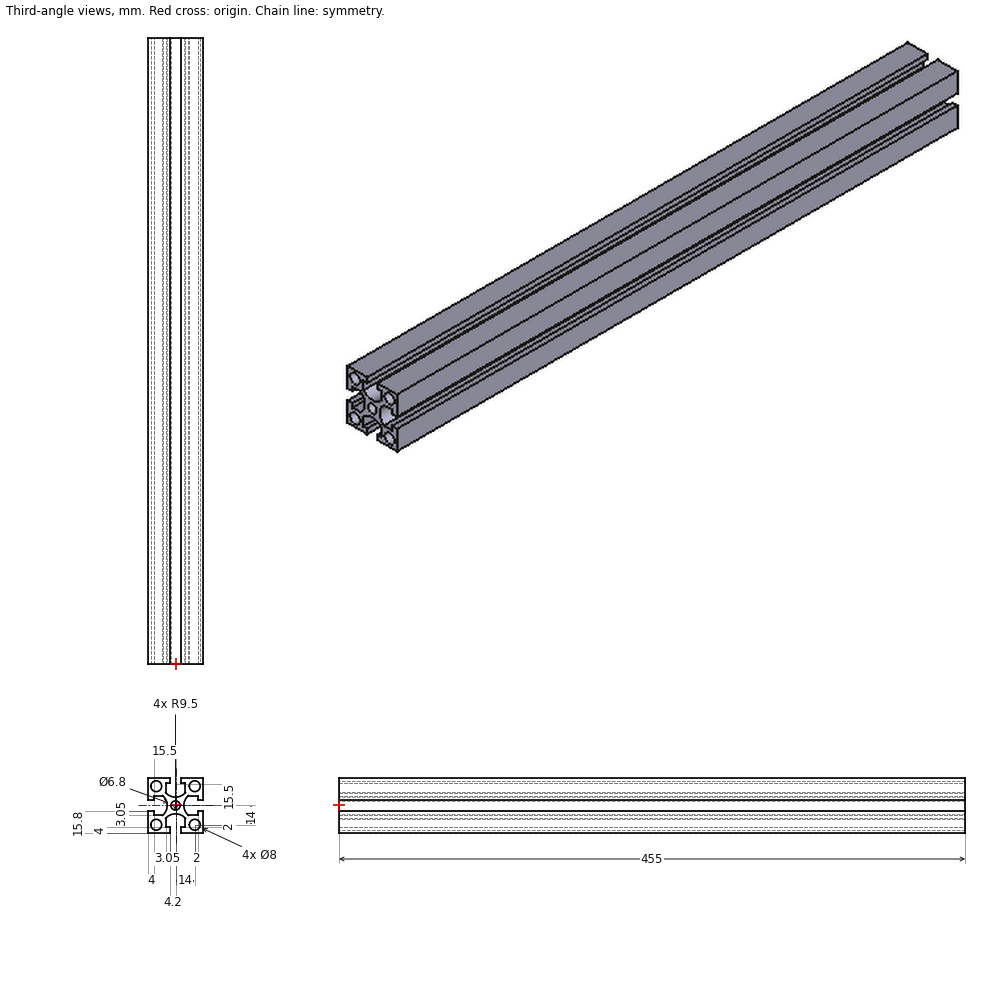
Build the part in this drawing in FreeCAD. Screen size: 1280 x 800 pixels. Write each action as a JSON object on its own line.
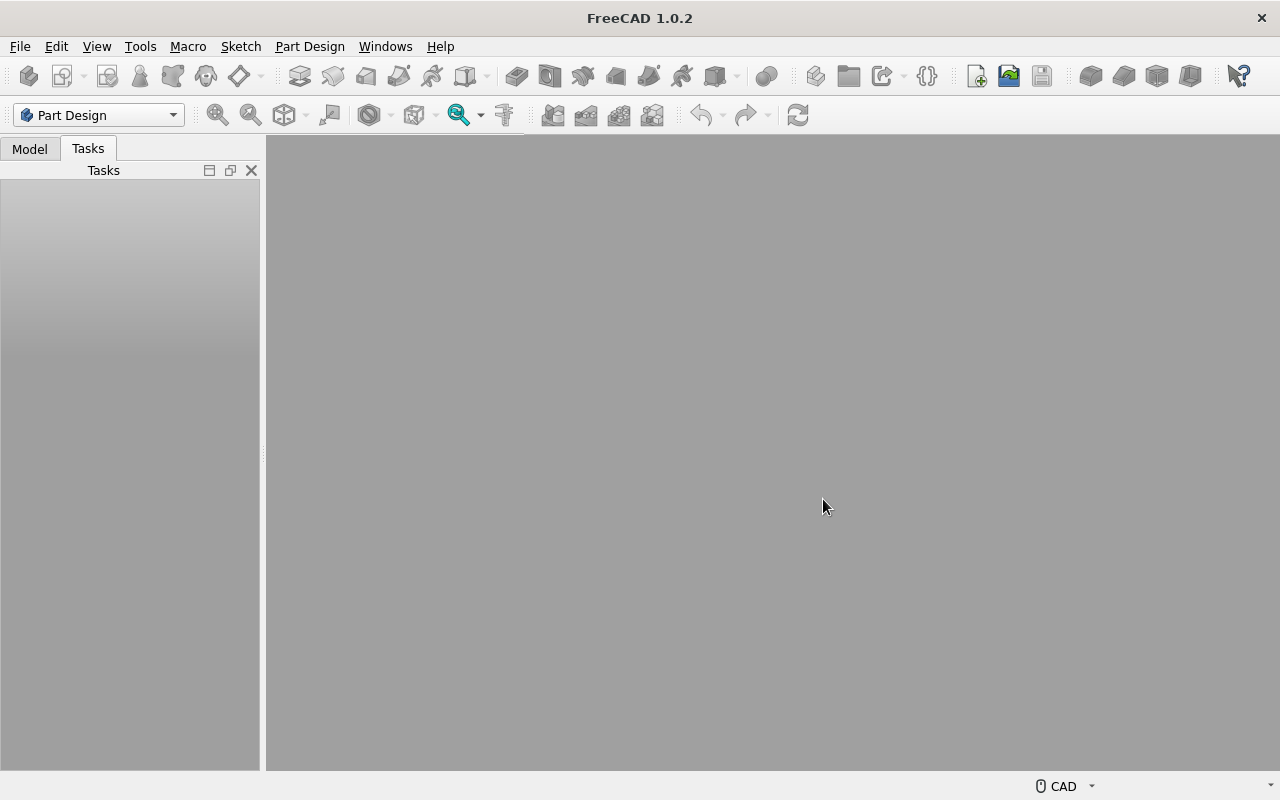
{"action": "left_click", "coordinate": [976, 76]}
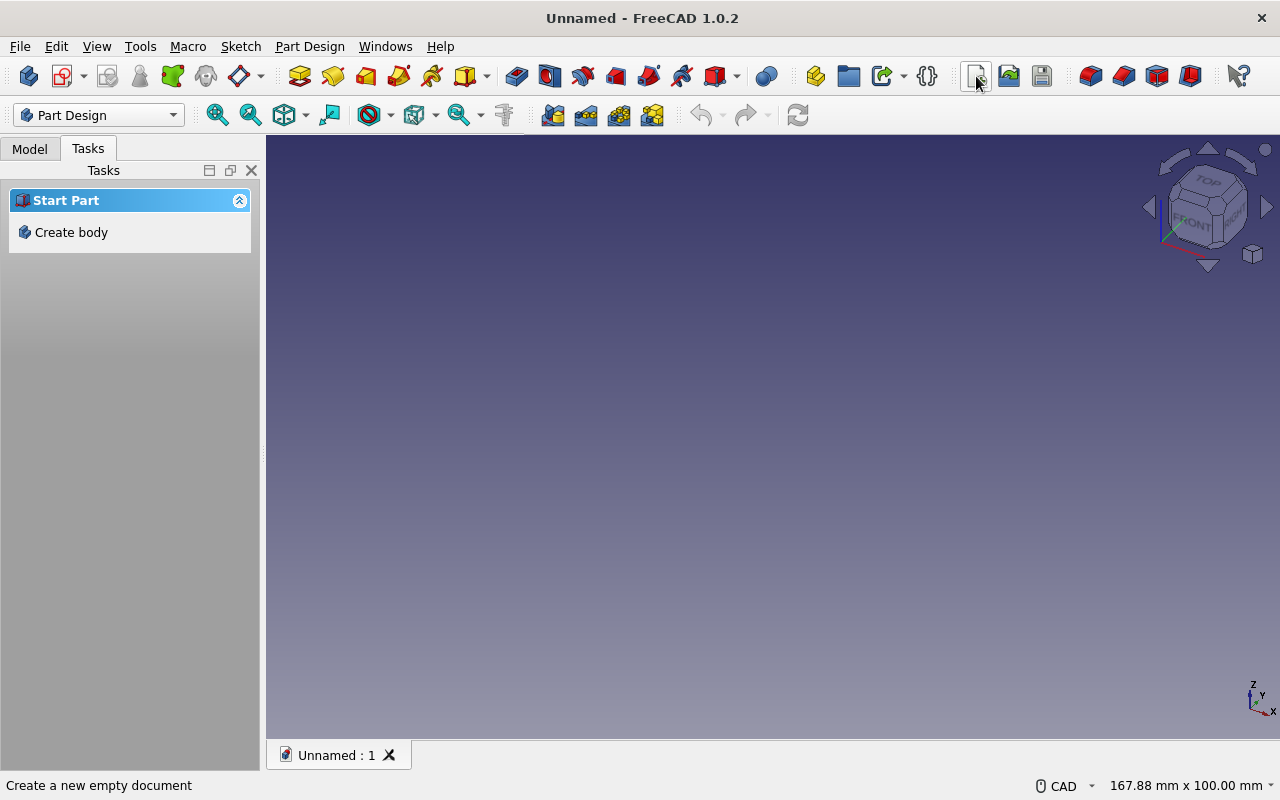
{"action": "left_click", "coordinate": [62, 76]}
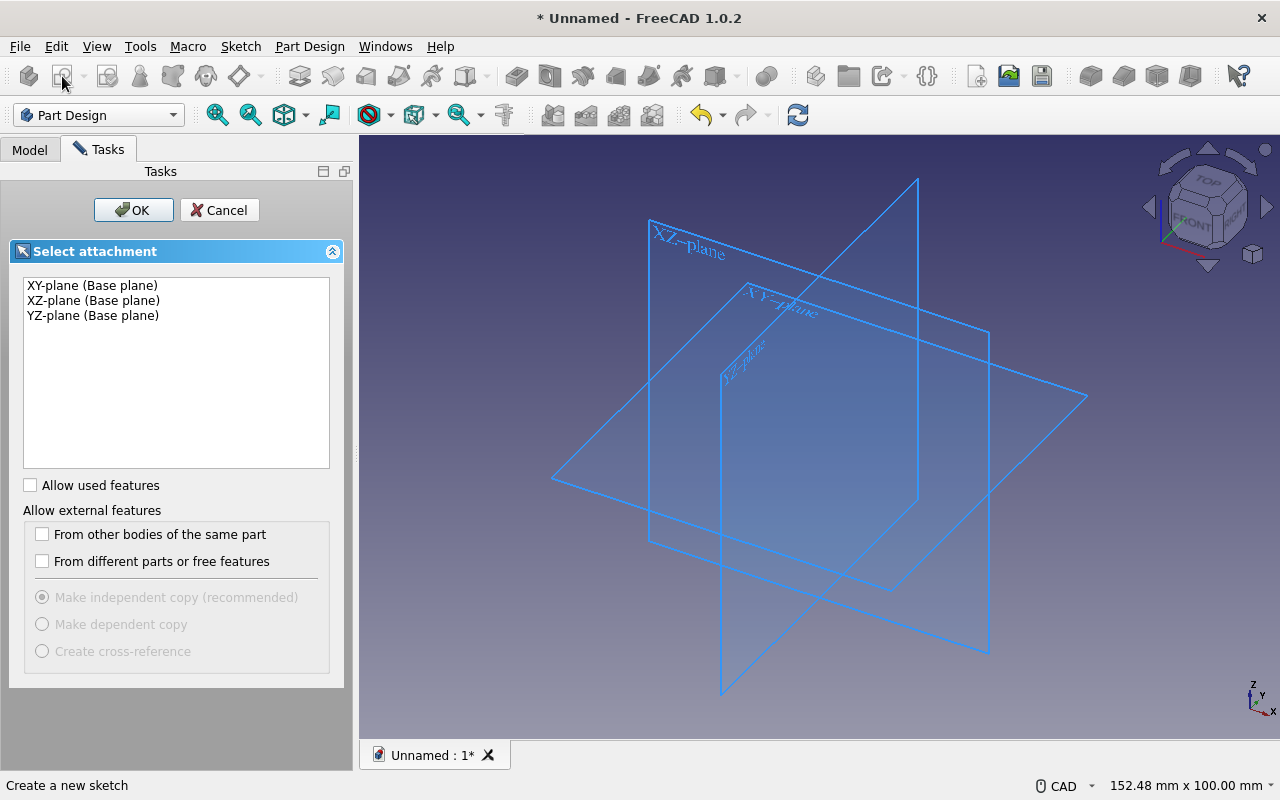
{"action": "left_click", "coordinate": [84, 300]}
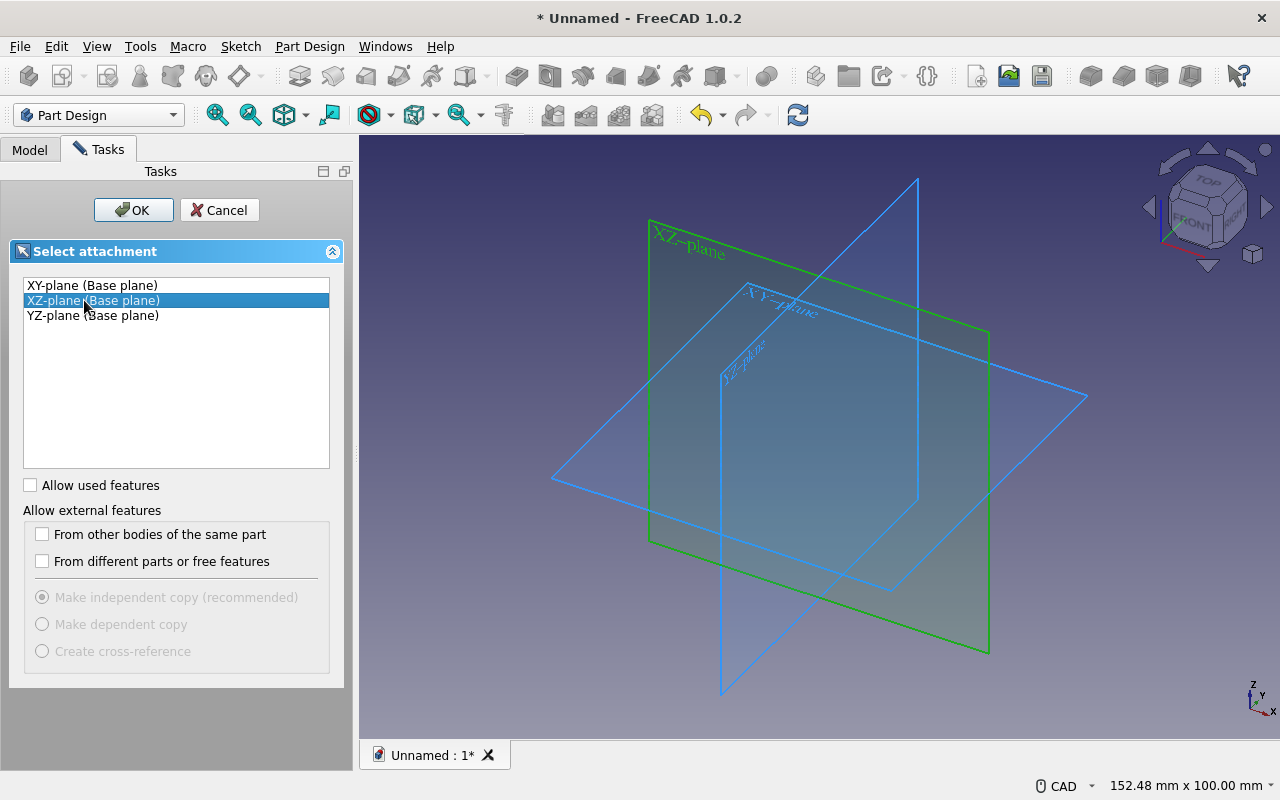
{"action": "left_click", "coordinate": [134, 210]}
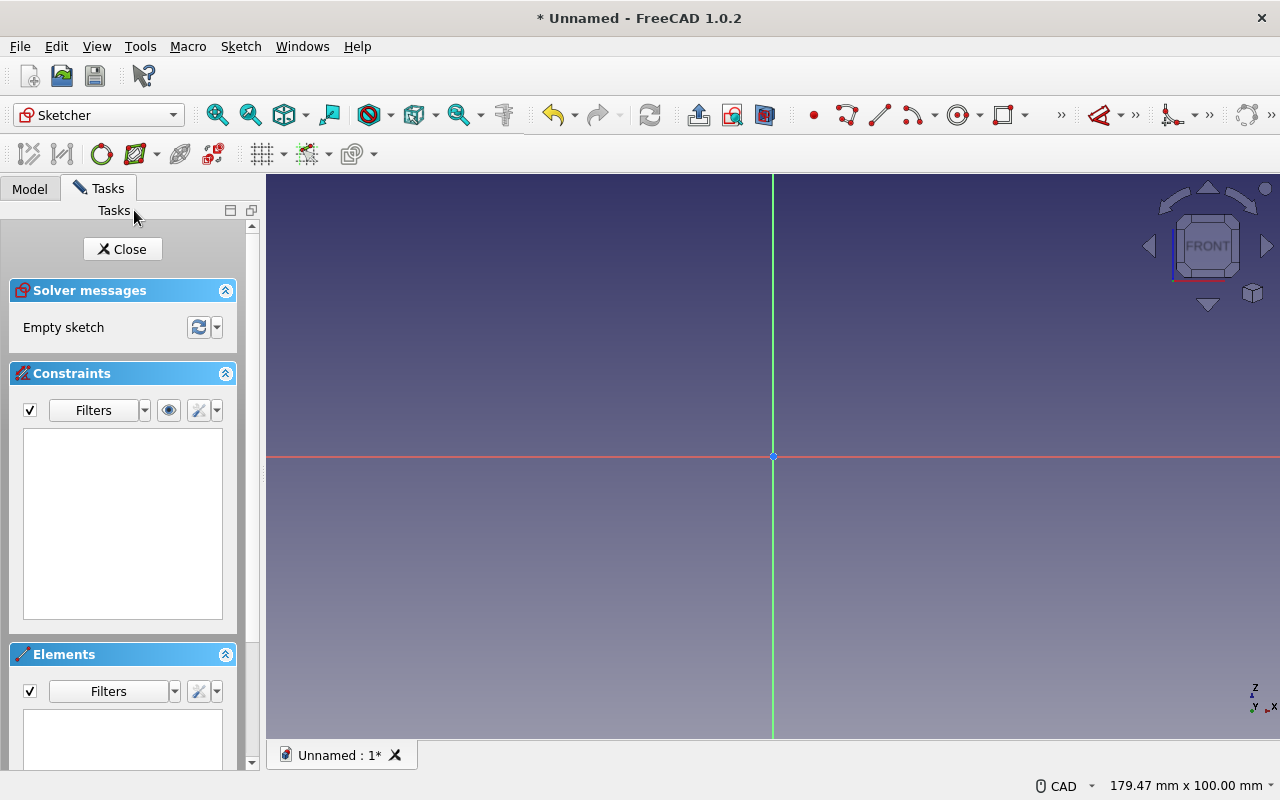
{"action": "scroll", "coordinate": [912, 456], "scroll_direction": "up", "scroll_amount": 2}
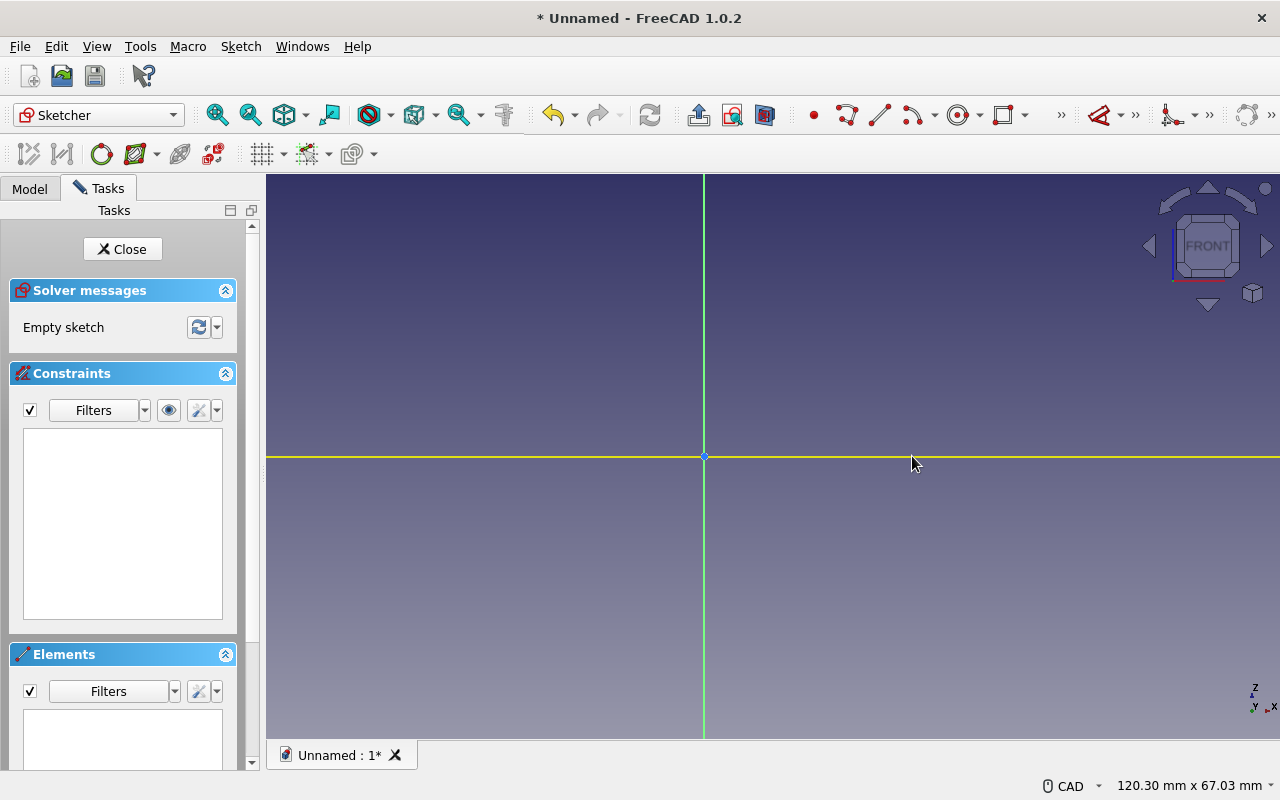
{"action": "left_click", "coordinate": [847, 116]}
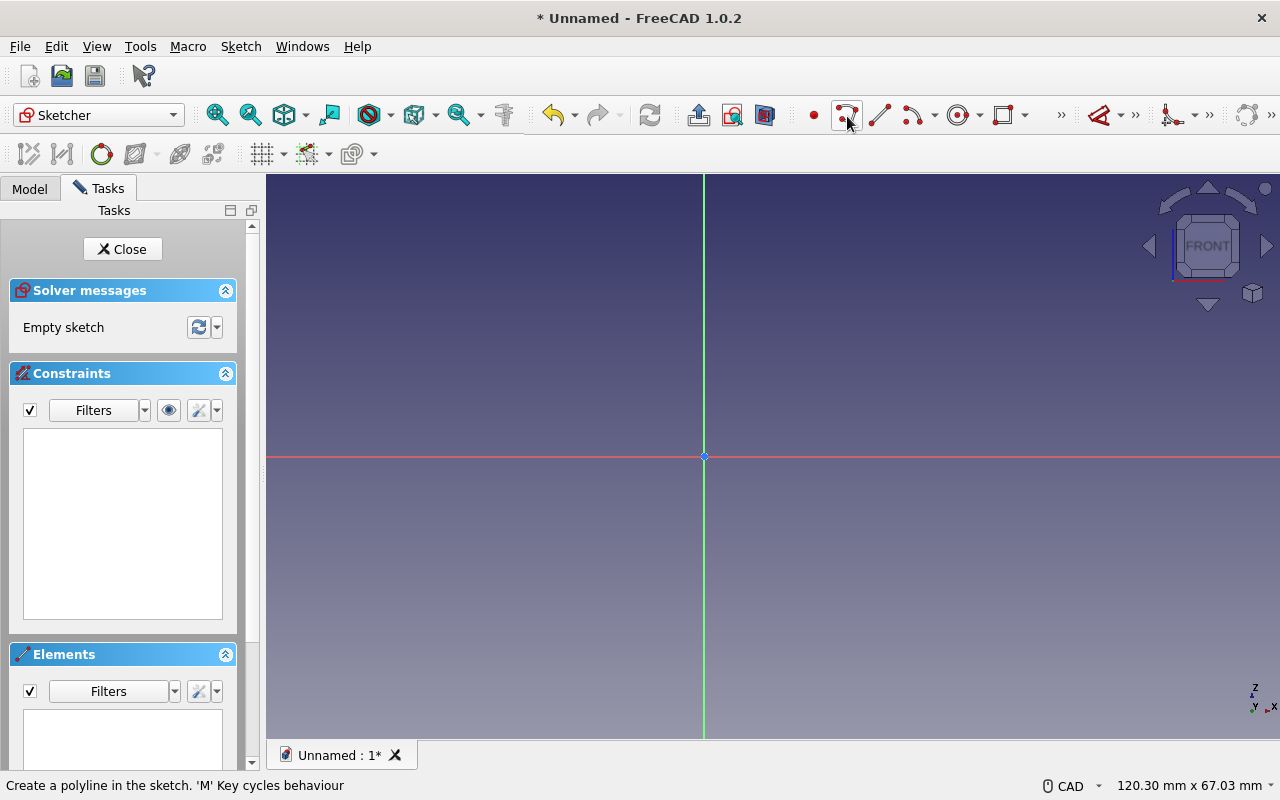
{"action": "left_click", "coordinate": [643, 535]}
{"action": "left_click", "coordinate": [643, 591]}
{"action": "left_click", "coordinate": [669, 591]}
{"action": "left_click", "coordinate": [669, 625]}
{"action": "left_click", "coordinate": [536, 625]}
{"action": "left_click", "coordinate": [536, 492]}
{"action": "left_click", "coordinate": [569, 492]}
{"action": "left_click", "coordinate": [569, 518]}
{"action": "left_click", "coordinate": [625, 518]}
{"action": "right_click", "coordinate": [625, 518]}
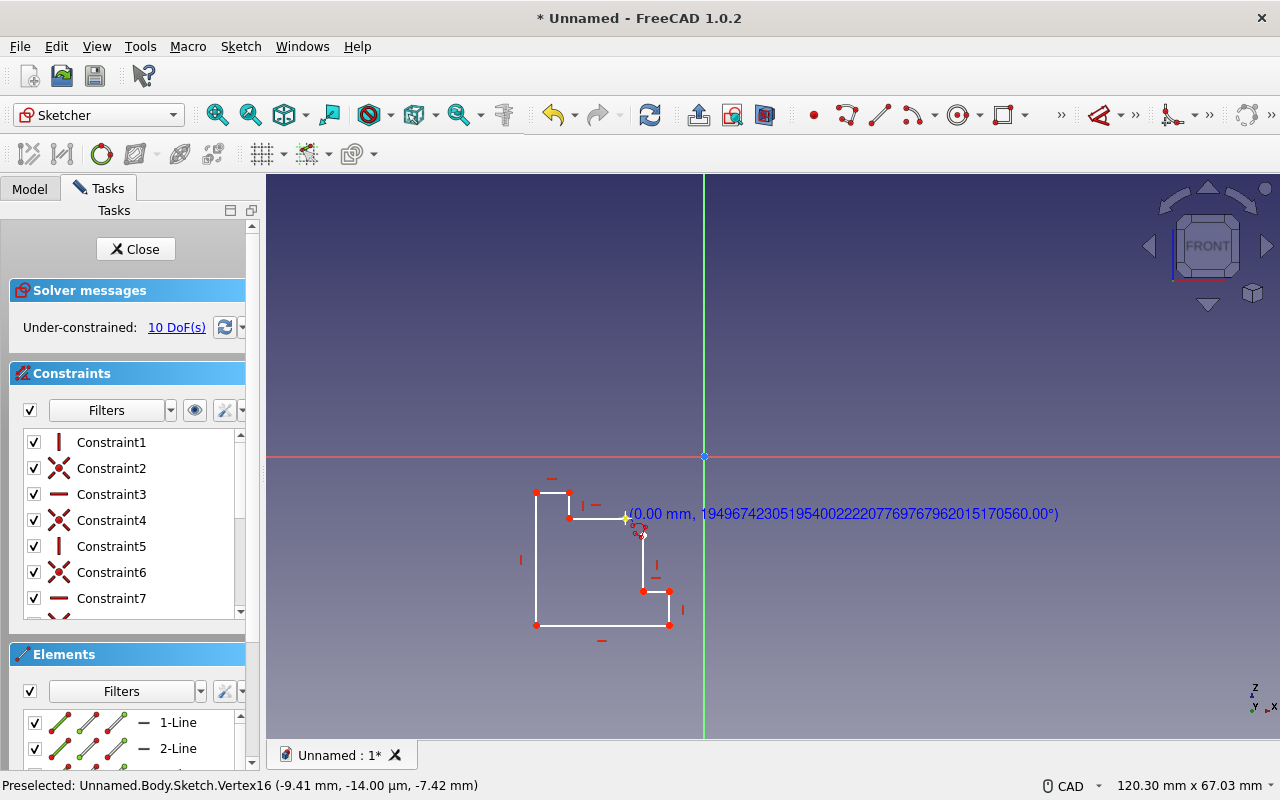
{"action": "left_click", "coordinate": [625, 395]}
{"action": "left_click", "coordinate": [569, 395]}
{"action": "left_click", "coordinate": [569, 421]}
{"action": "left_click", "coordinate": [536, 421]}
{"action": "left_click", "coordinate": [536, 288]}
{"action": "left_click", "coordinate": [669, 288]}
{"action": "left_click", "coordinate": [669, 322]}
{"action": "left_click", "coordinate": [643, 322]}
{"action": "left_click", "coordinate": [643, 378]}
{"action": "right_click", "coordinate": [643, 378]}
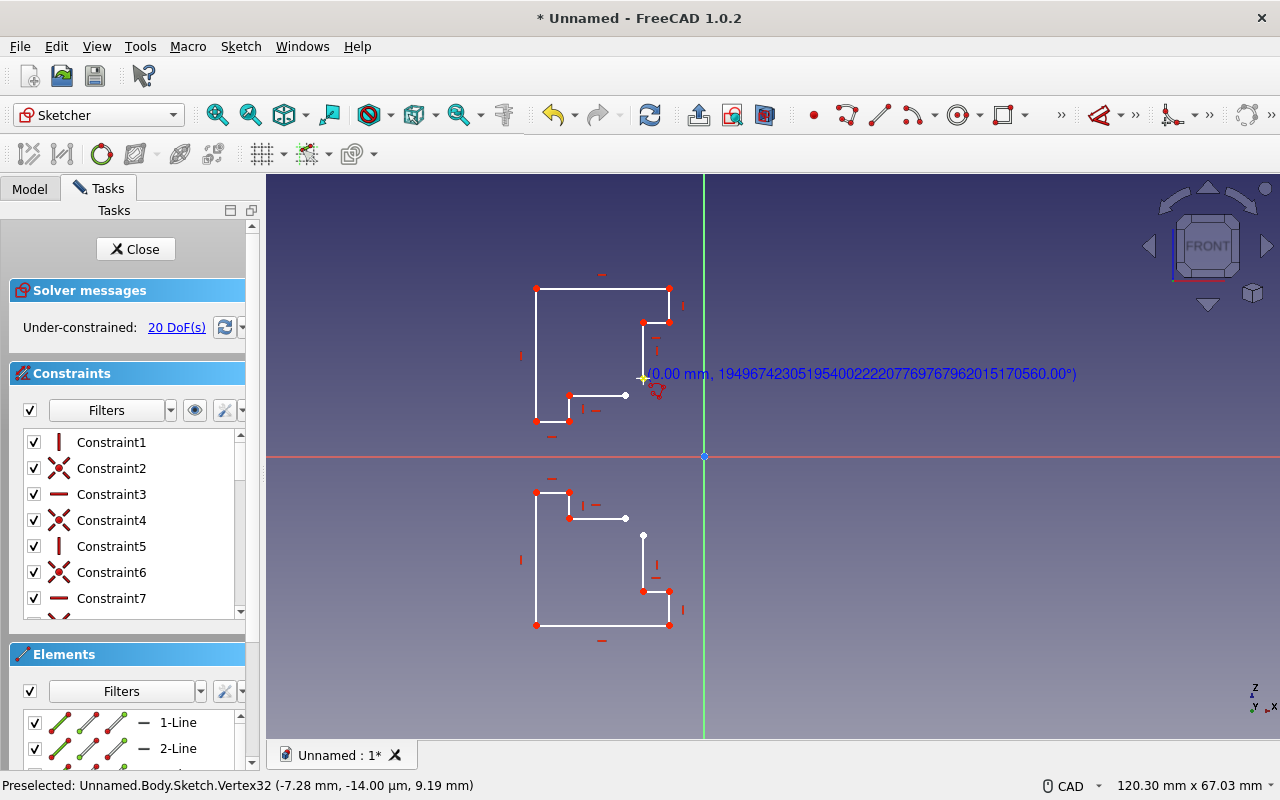
{"action": "left_click", "coordinate": [765, 378]}
{"action": "left_click", "coordinate": [765, 322]}
{"action": "left_click", "coordinate": [740, 322]}
{"action": "left_click", "coordinate": [740, 288]}
{"action": "left_click", "coordinate": [873, 288]}
{"action": "left_click", "coordinate": [873, 421]}
{"action": "left_click", "coordinate": [839, 421]}
{"action": "left_click", "coordinate": [839, 395]}
{"action": "left_click", "coordinate": [783, 395]}
{"action": "right_click", "coordinate": [783, 395]}